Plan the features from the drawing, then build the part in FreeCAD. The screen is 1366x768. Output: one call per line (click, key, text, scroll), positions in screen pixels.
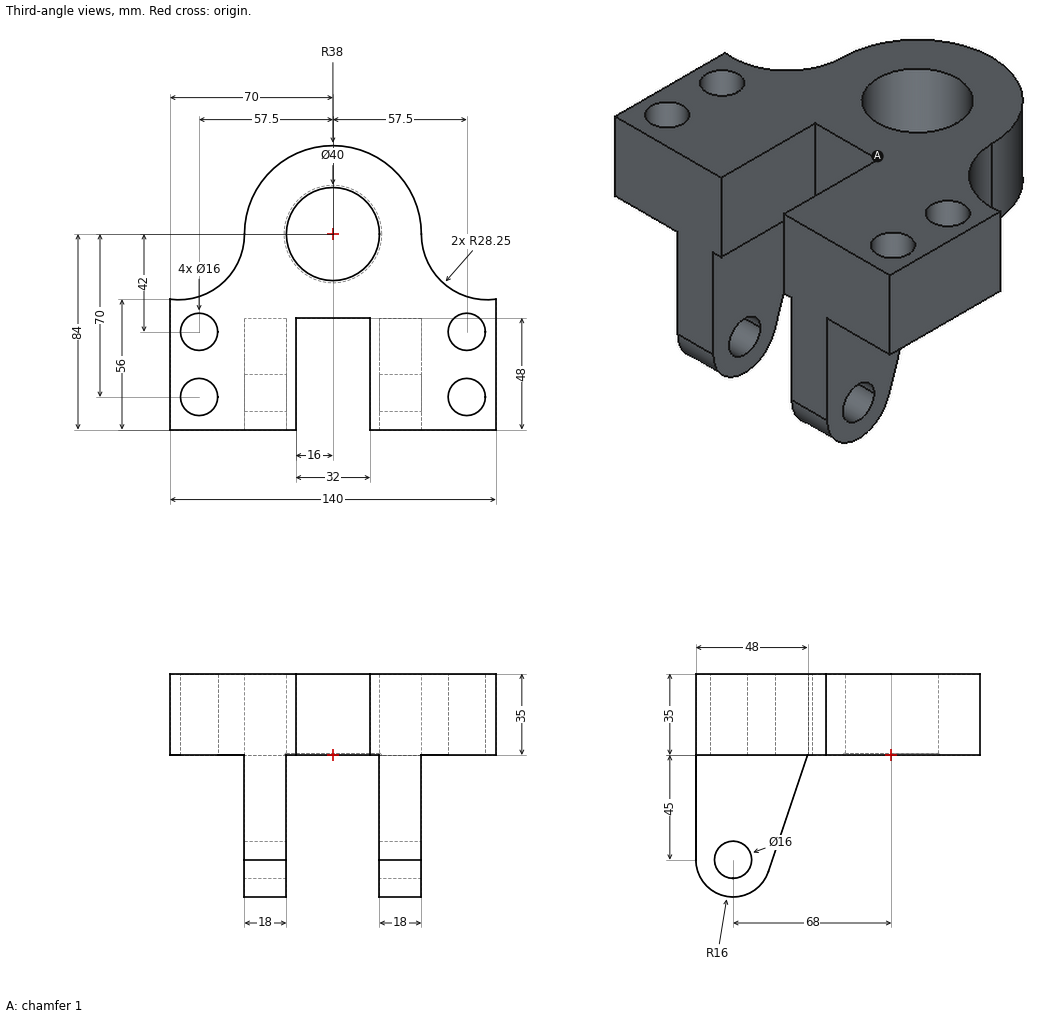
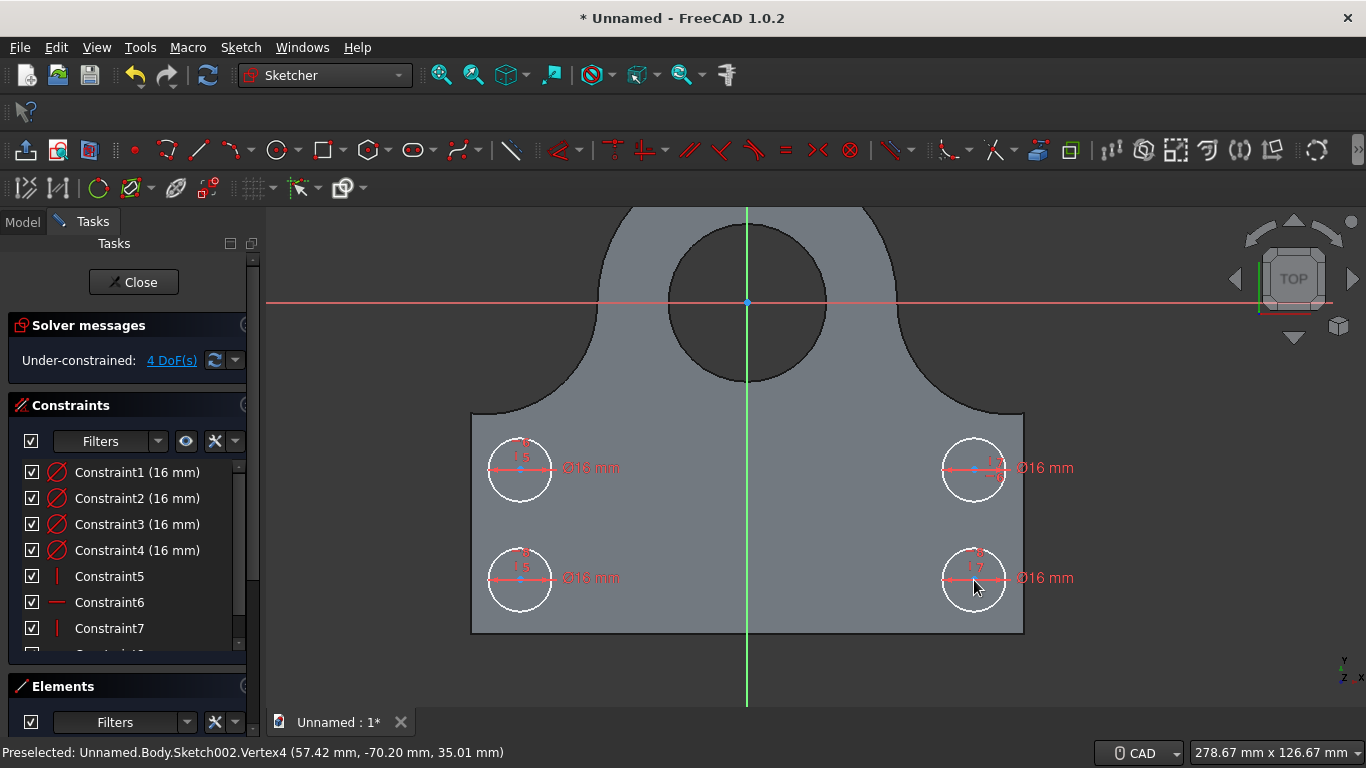
key(d)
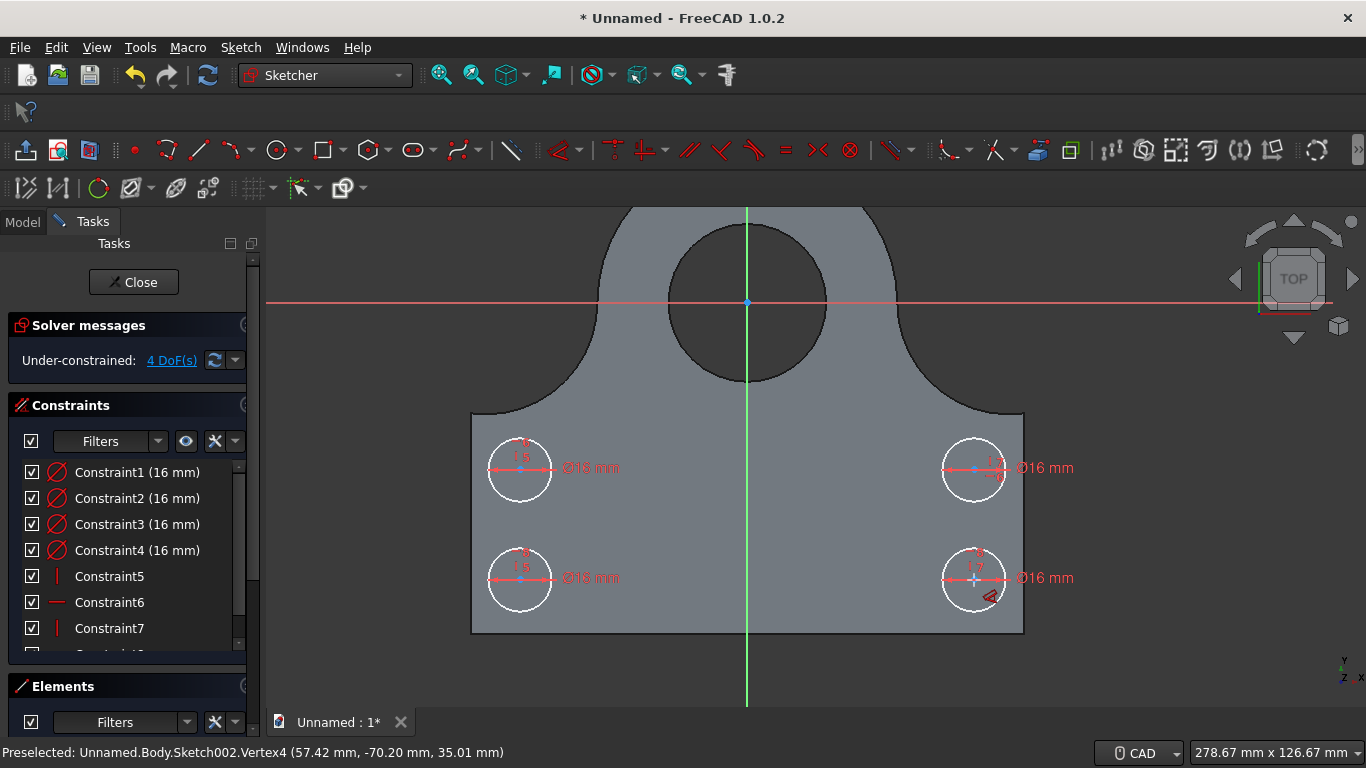
click(520, 470)
click(486, 386)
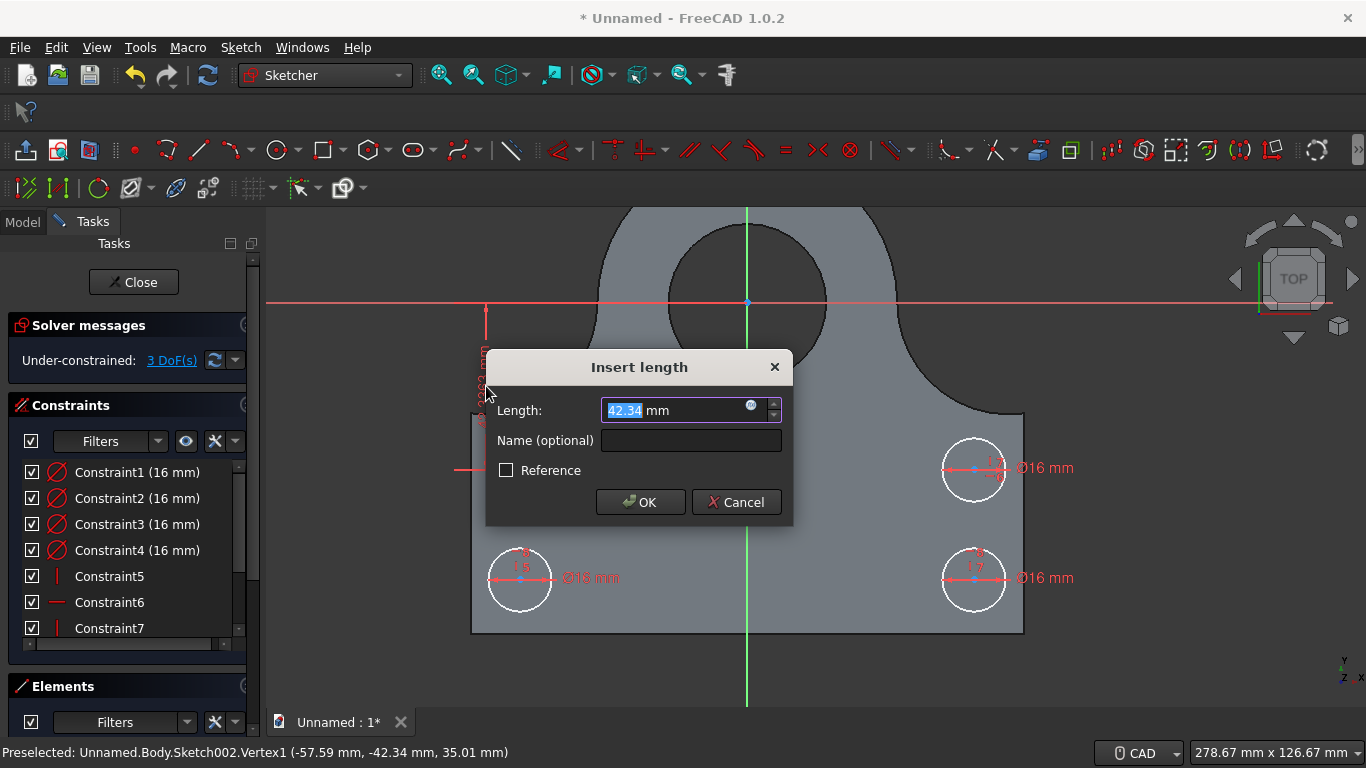
text(42)
key(Return)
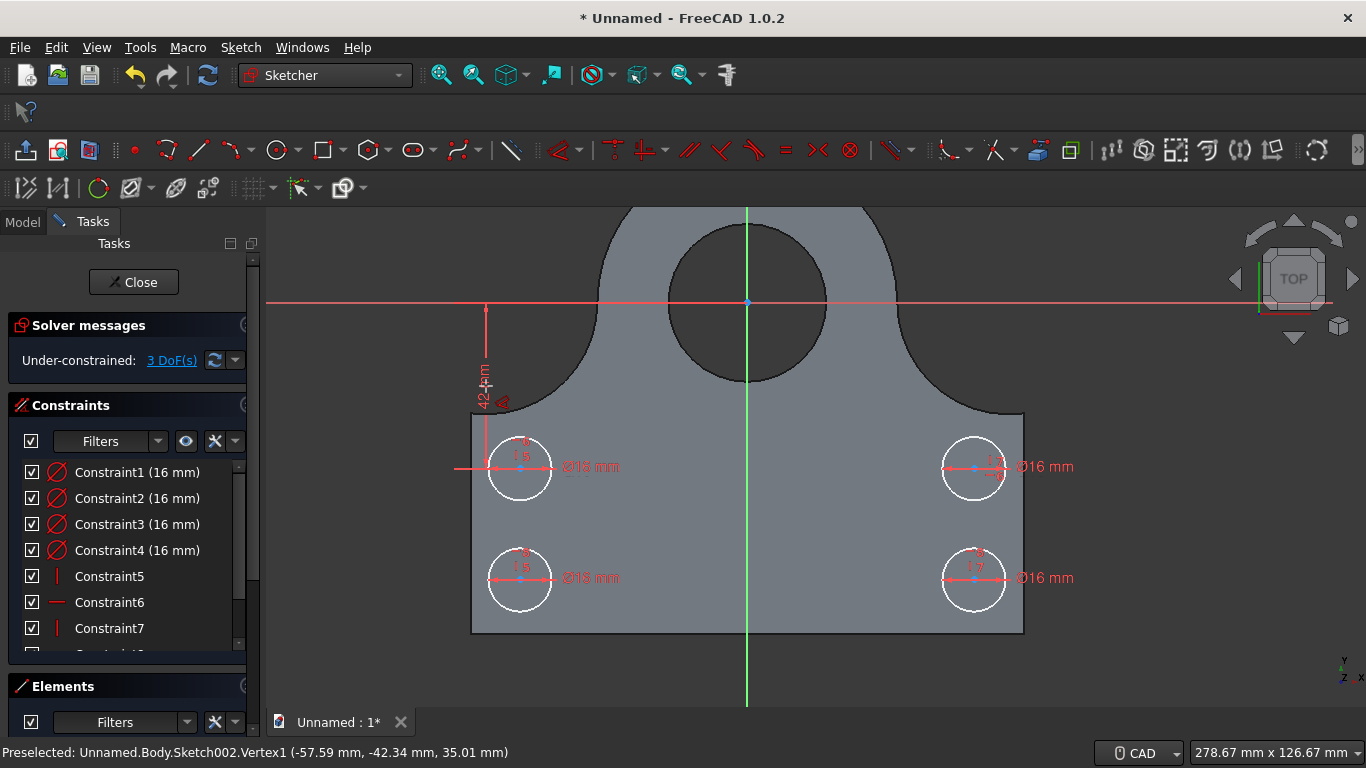
click(520, 580)
click(486, 505)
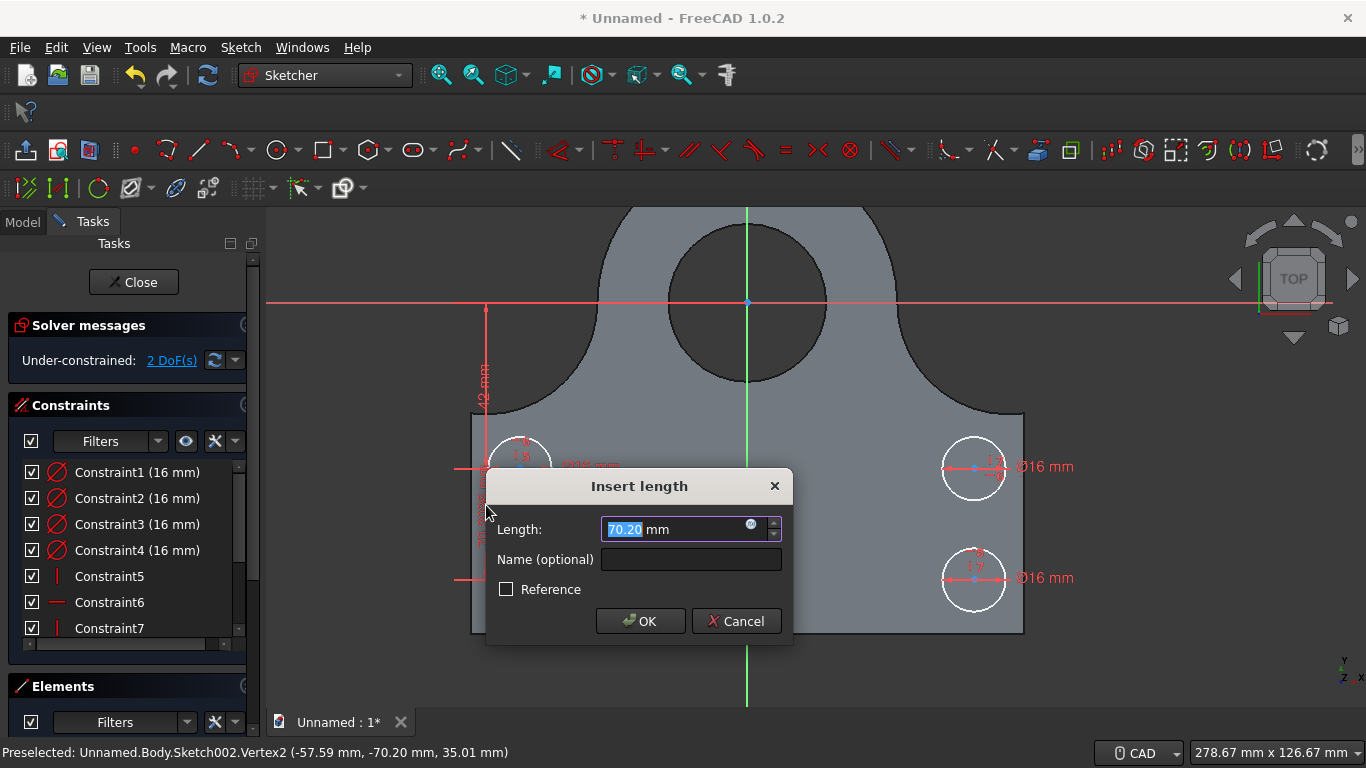
text(70)
key(Return)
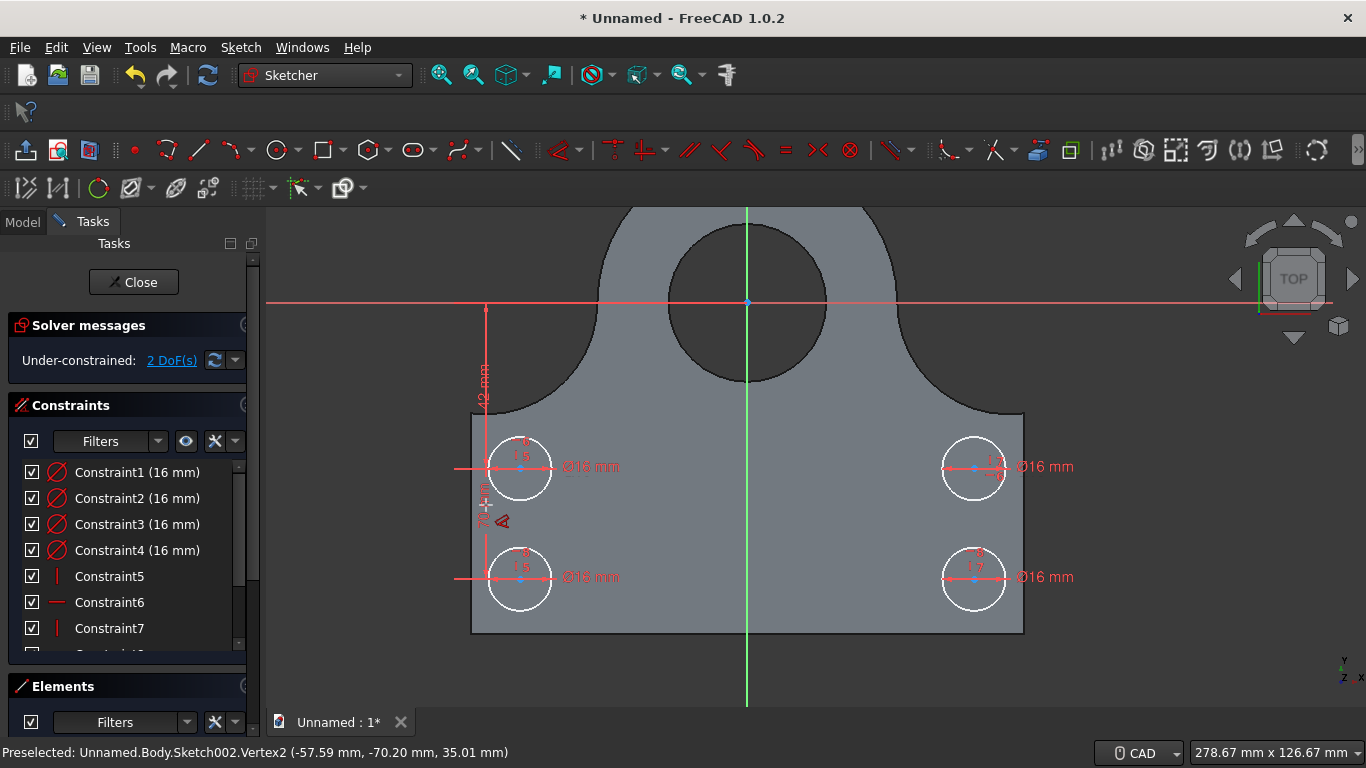
click(520, 469)
click(634, 269)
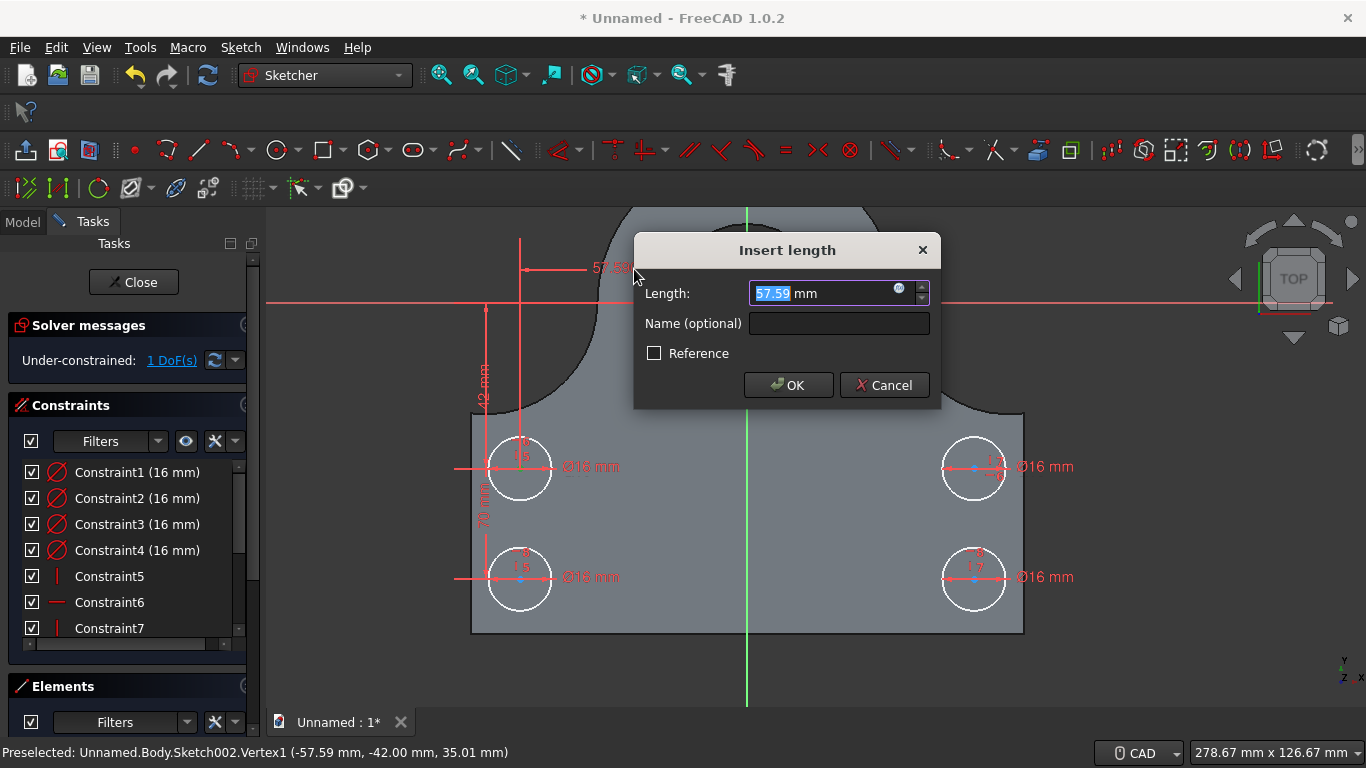
text(57.5)
key(Return)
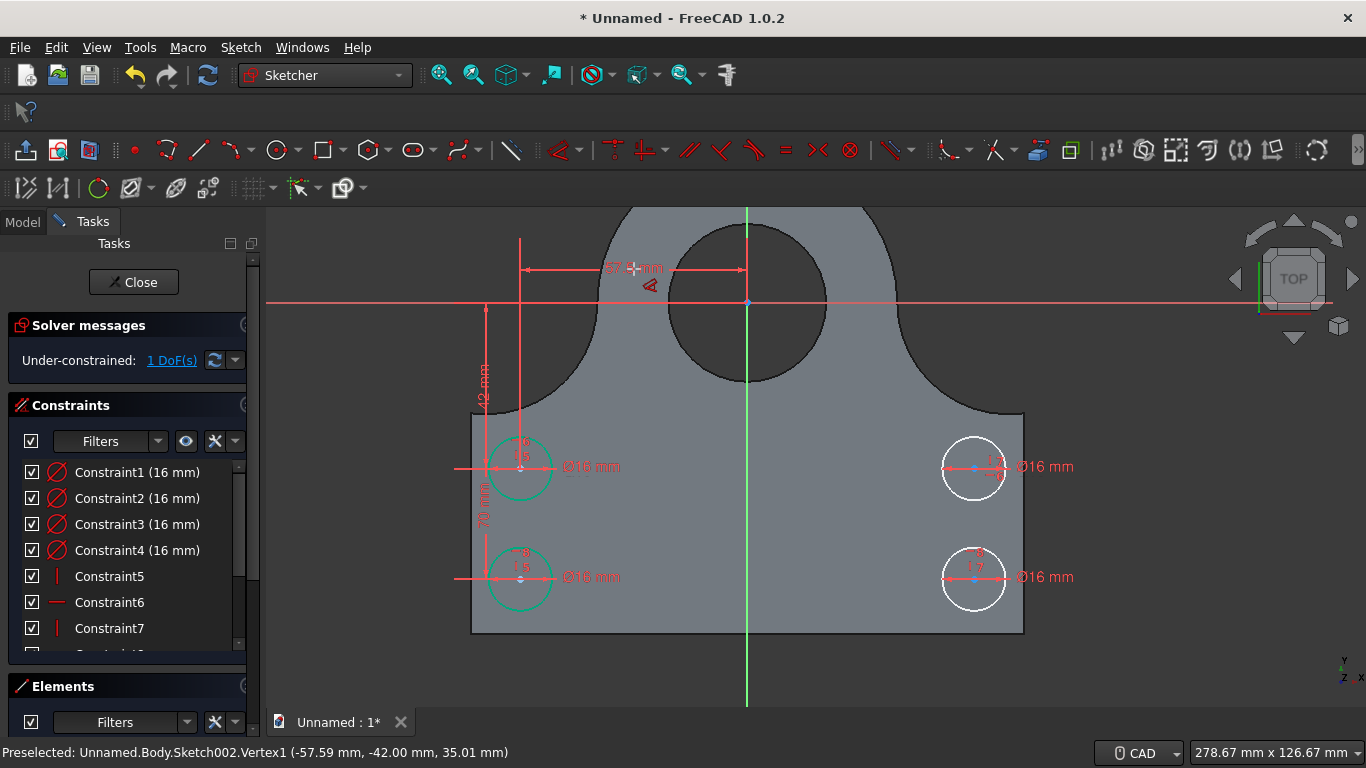
click(974, 469)
click(861, 269)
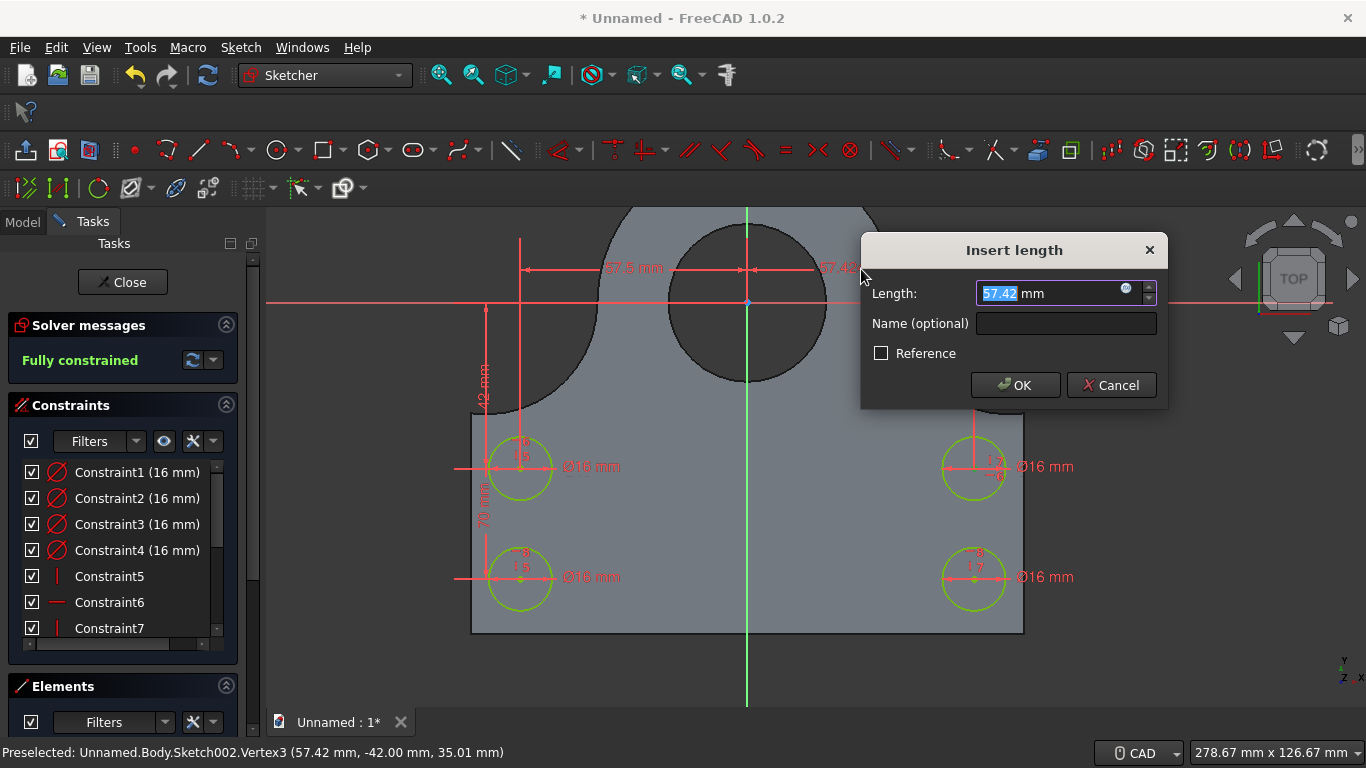
text(57.5)
key(Return)
key(Escape)